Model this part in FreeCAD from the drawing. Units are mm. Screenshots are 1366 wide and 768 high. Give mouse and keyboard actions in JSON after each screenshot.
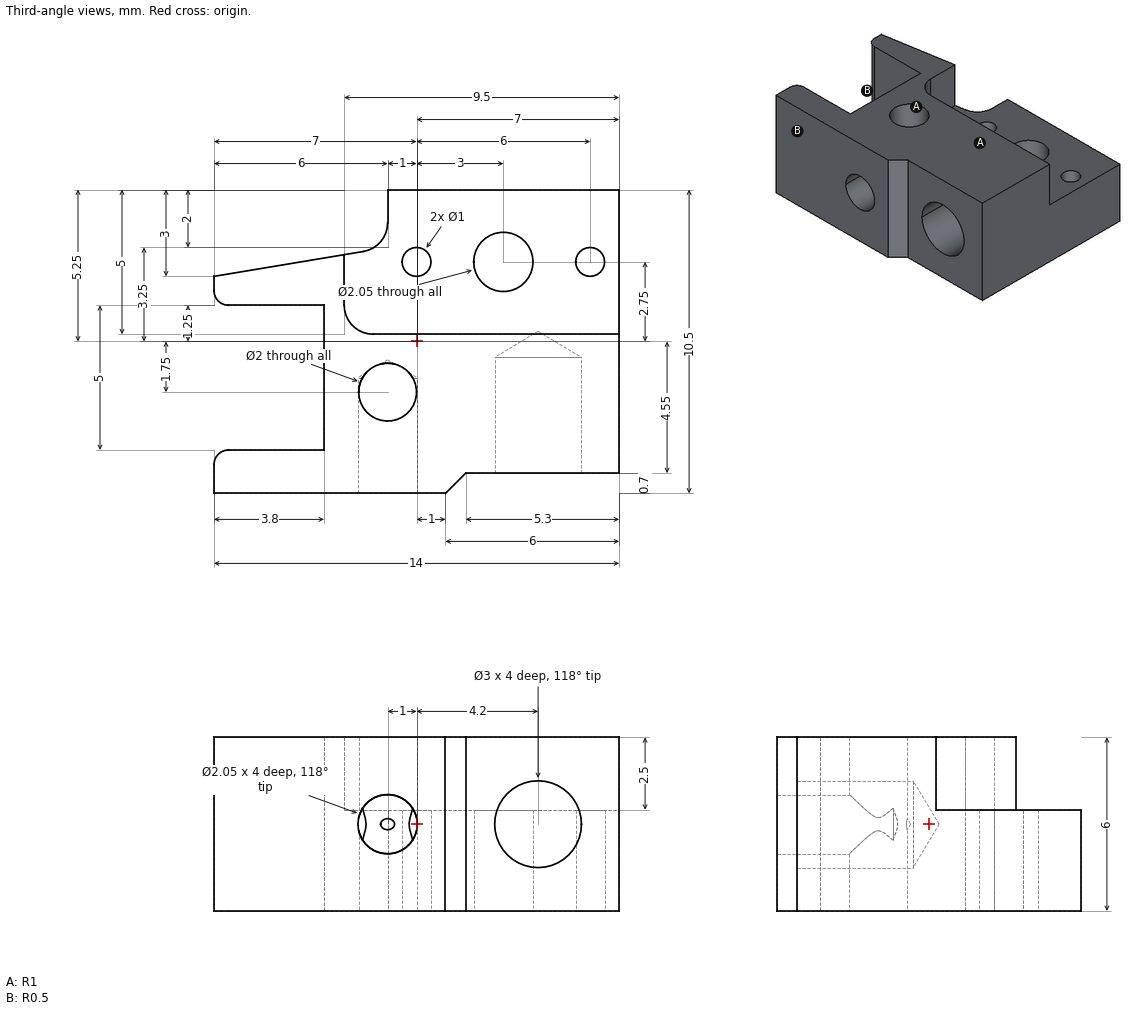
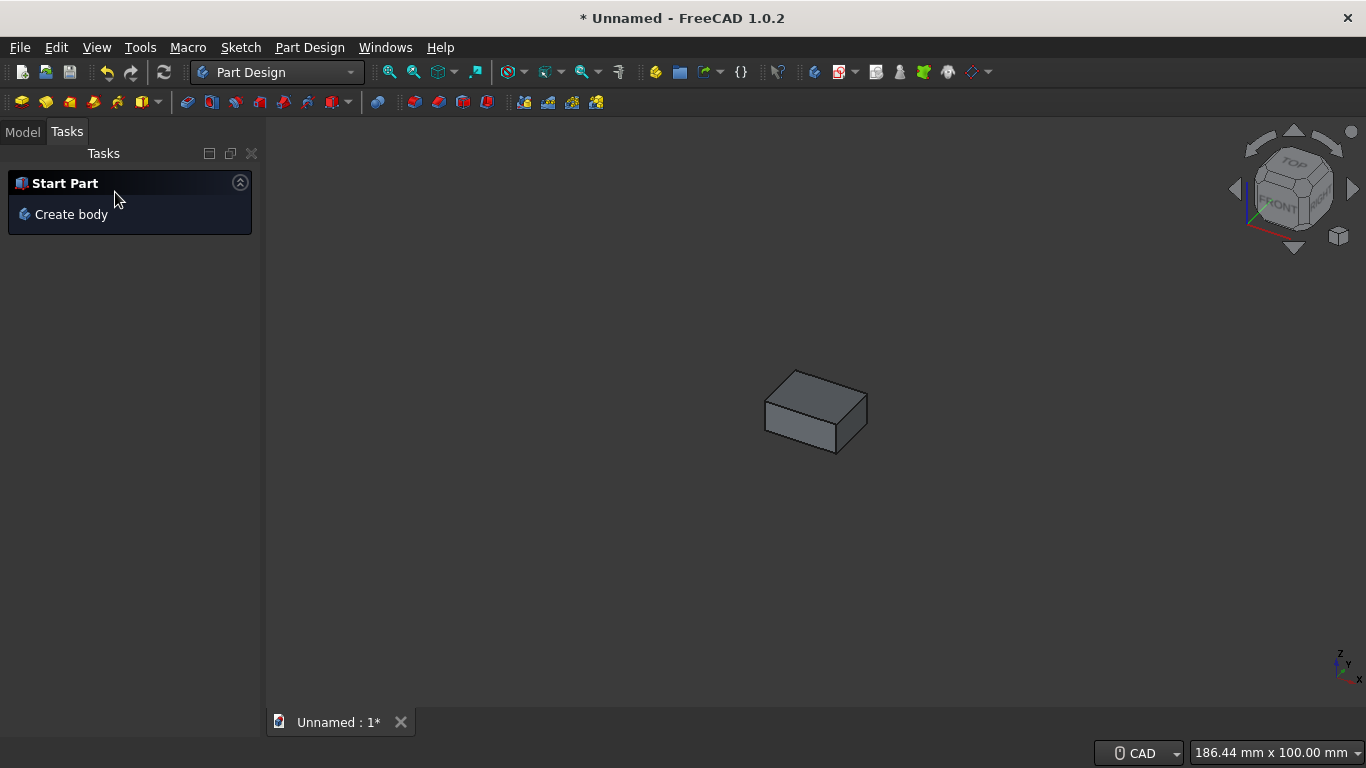
{"action": "left_click", "coordinate": [390, 72]}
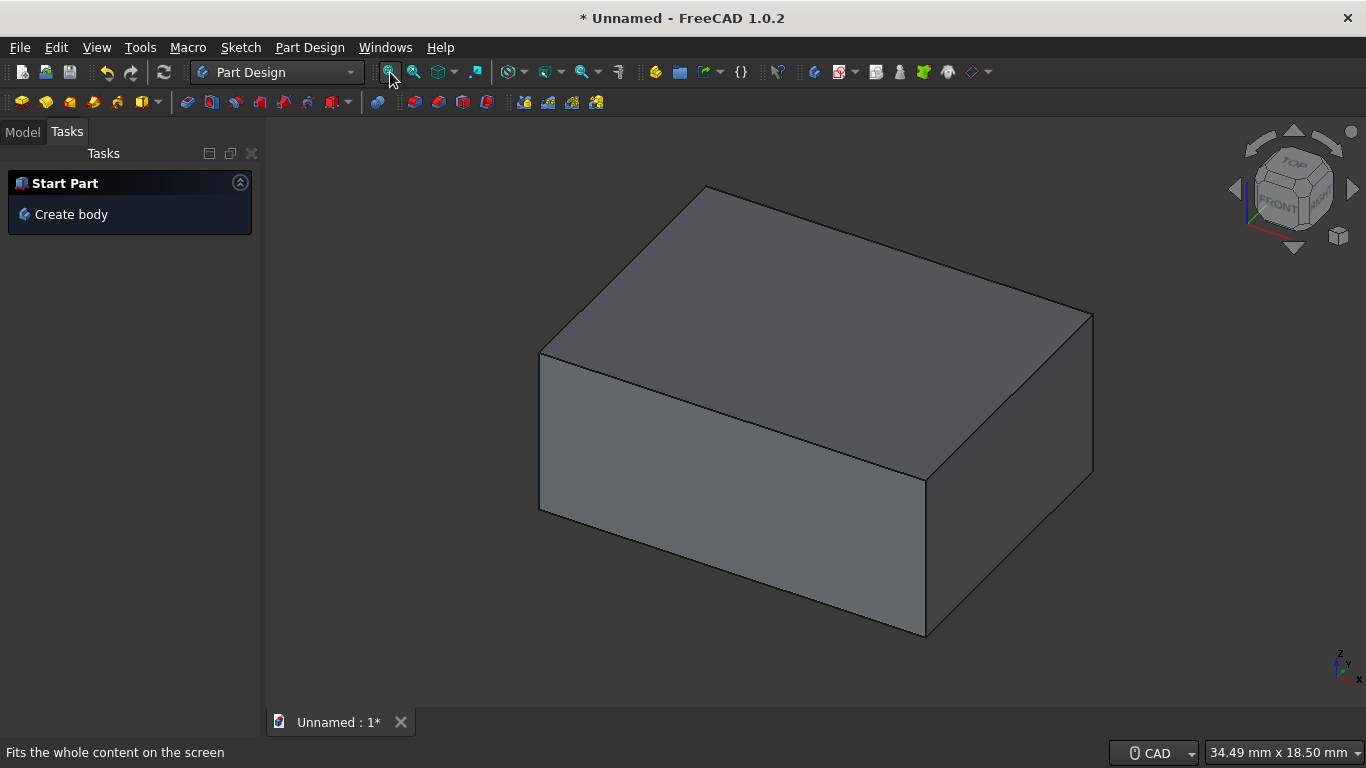
{"action": "left_click", "coordinate": [816, 333]}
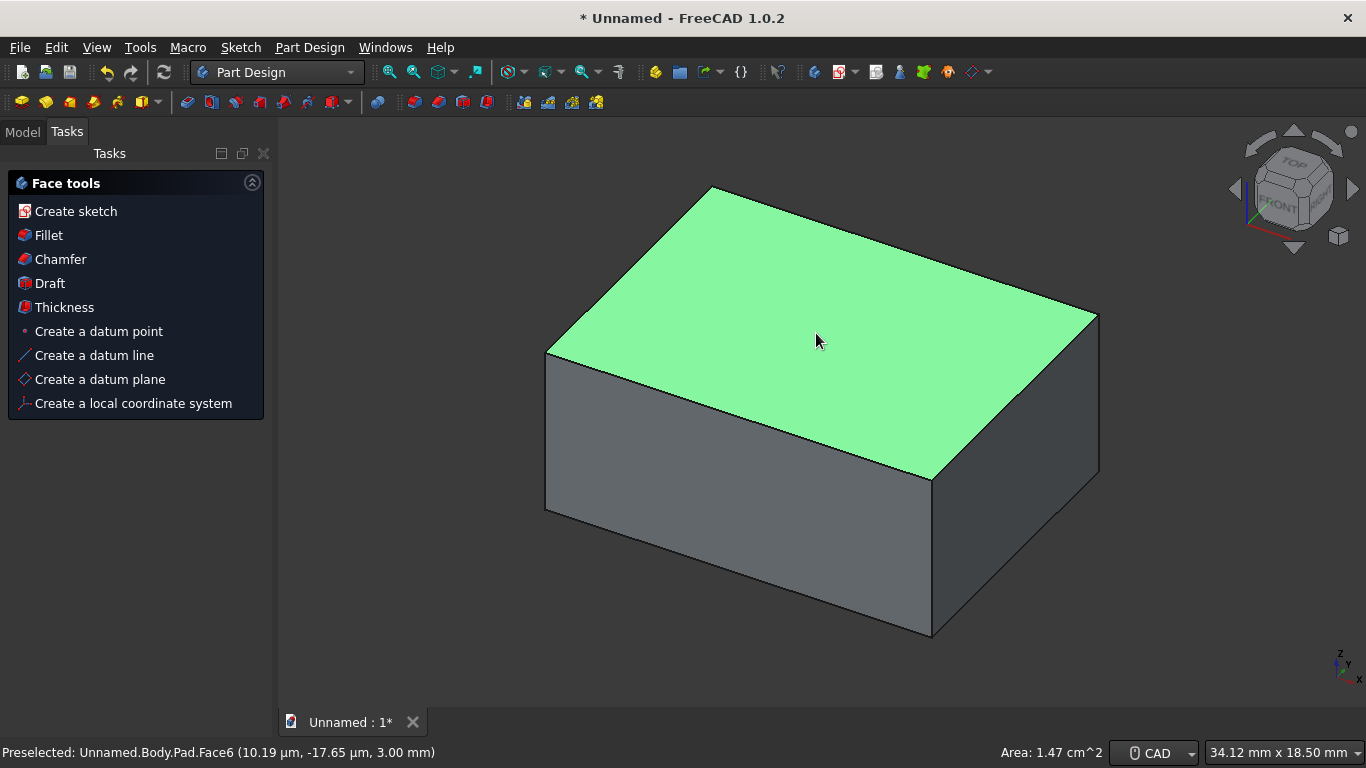
{"action": "left_click", "coordinate": [840, 72]}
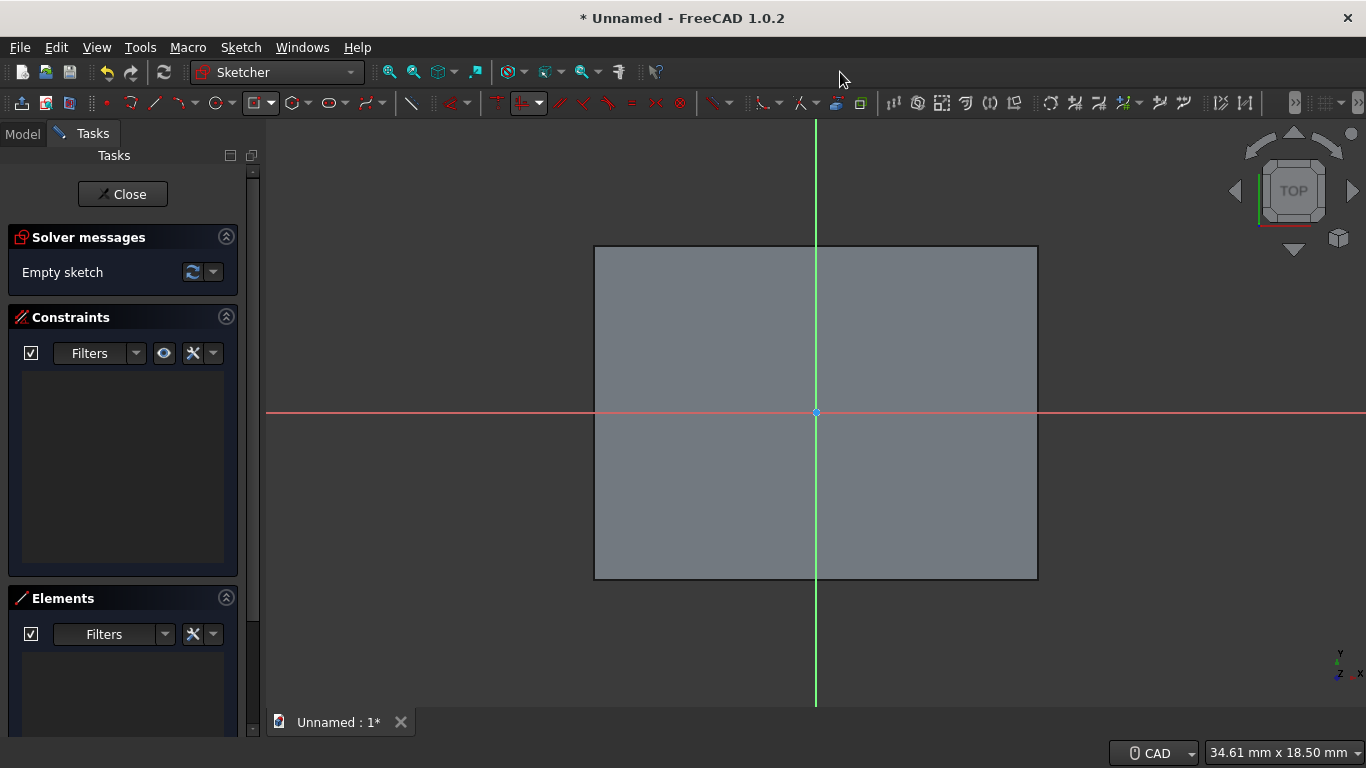
{"action": "scroll", "coordinate": [1002, 261], "scroll_direction": "up", "scroll_amount": 4}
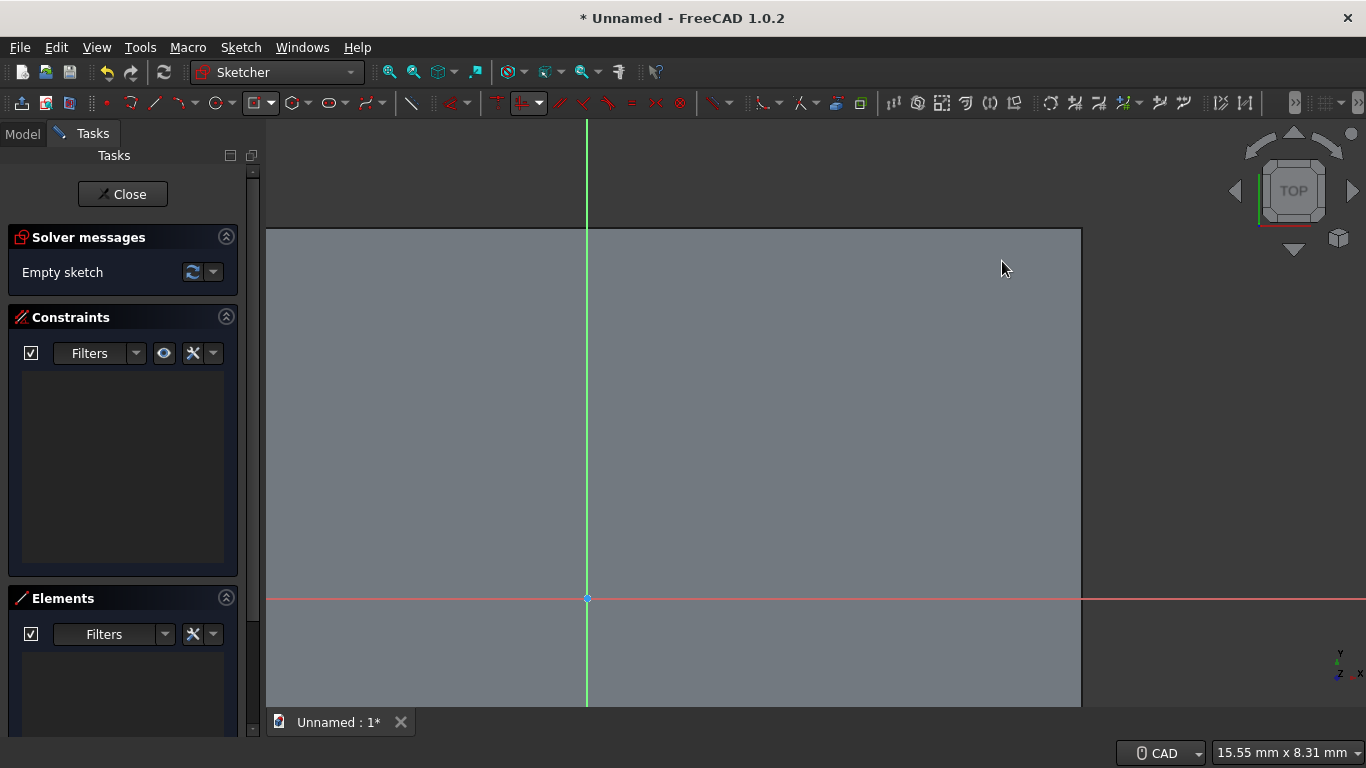
{"action": "left_click", "coordinate": [274, 104]}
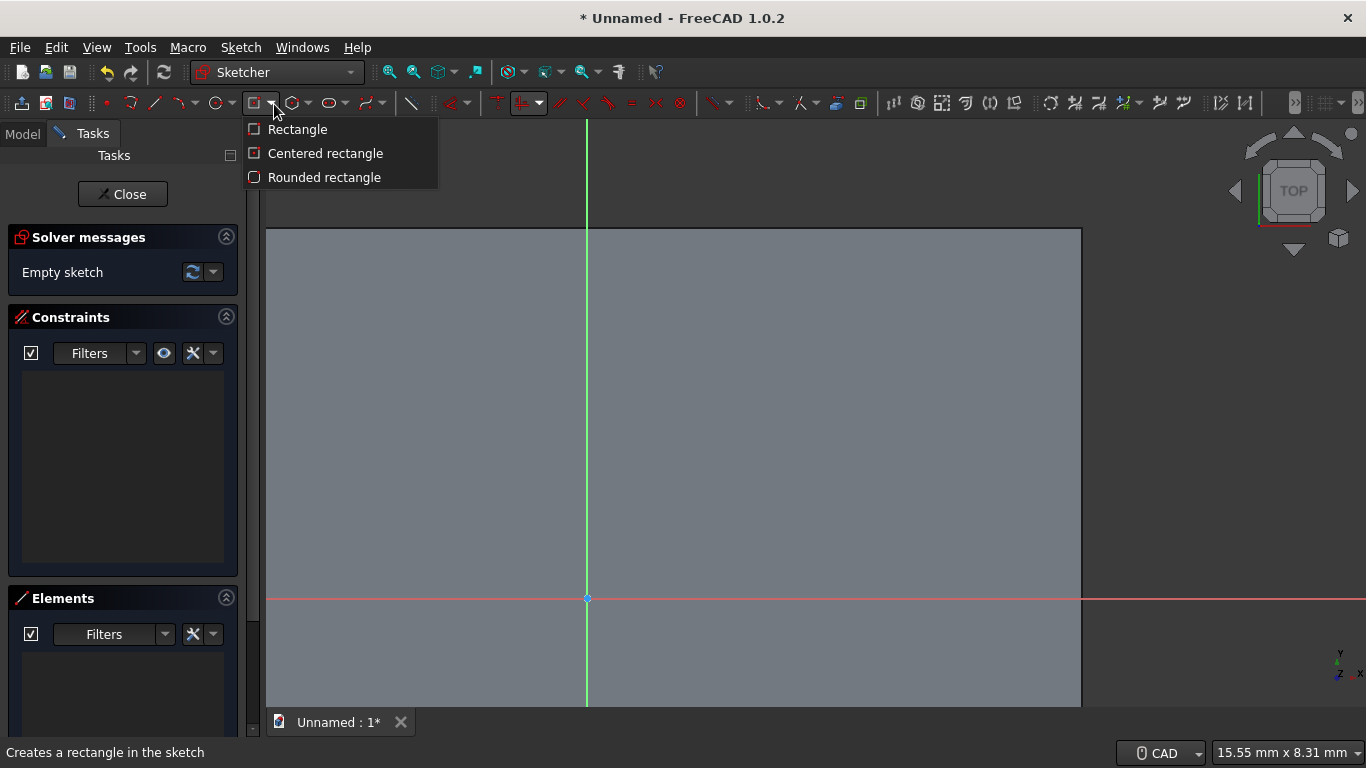
{"action": "left_click", "coordinate": [340, 129]}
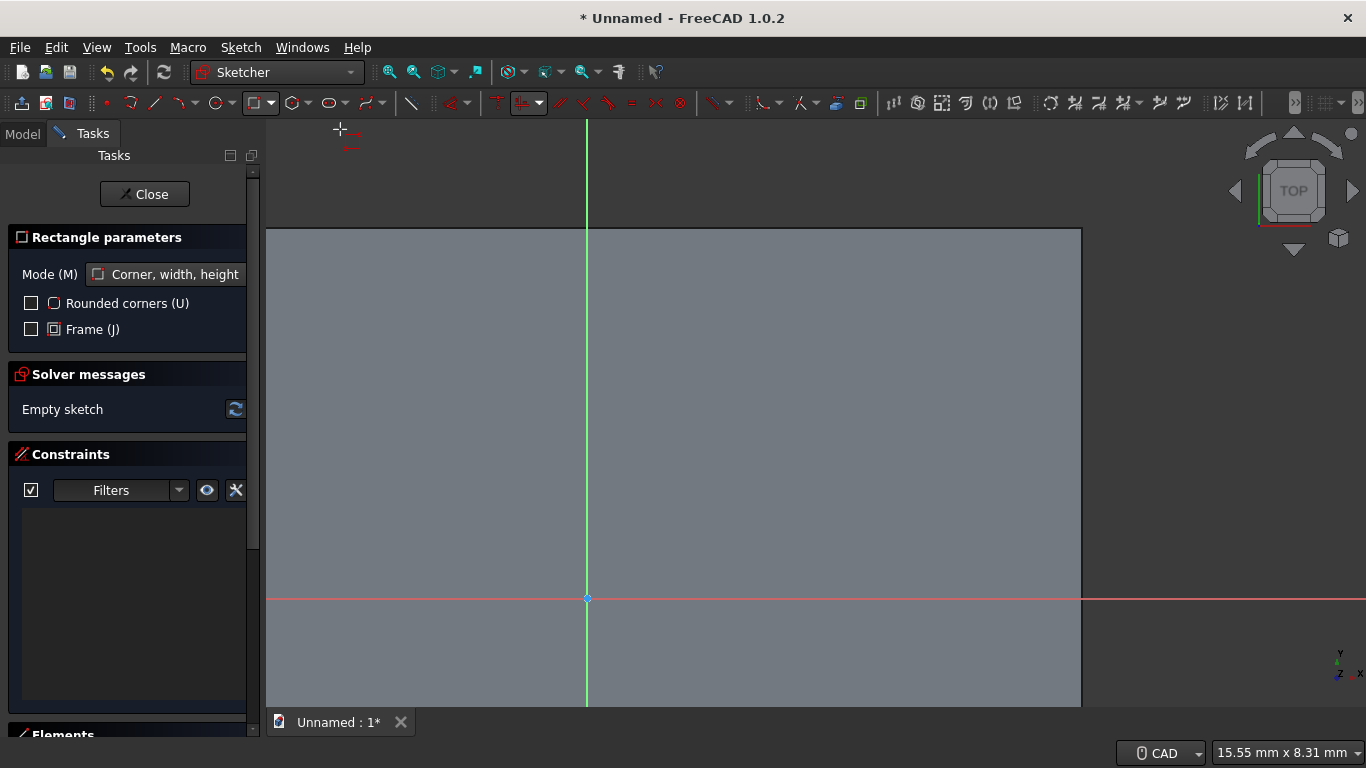
{"action": "left_click", "coordinate": [410, 228]}
{"action": "left_click", "coordinate": [1082, 581]}
{"action": "key", "text": "Escape"}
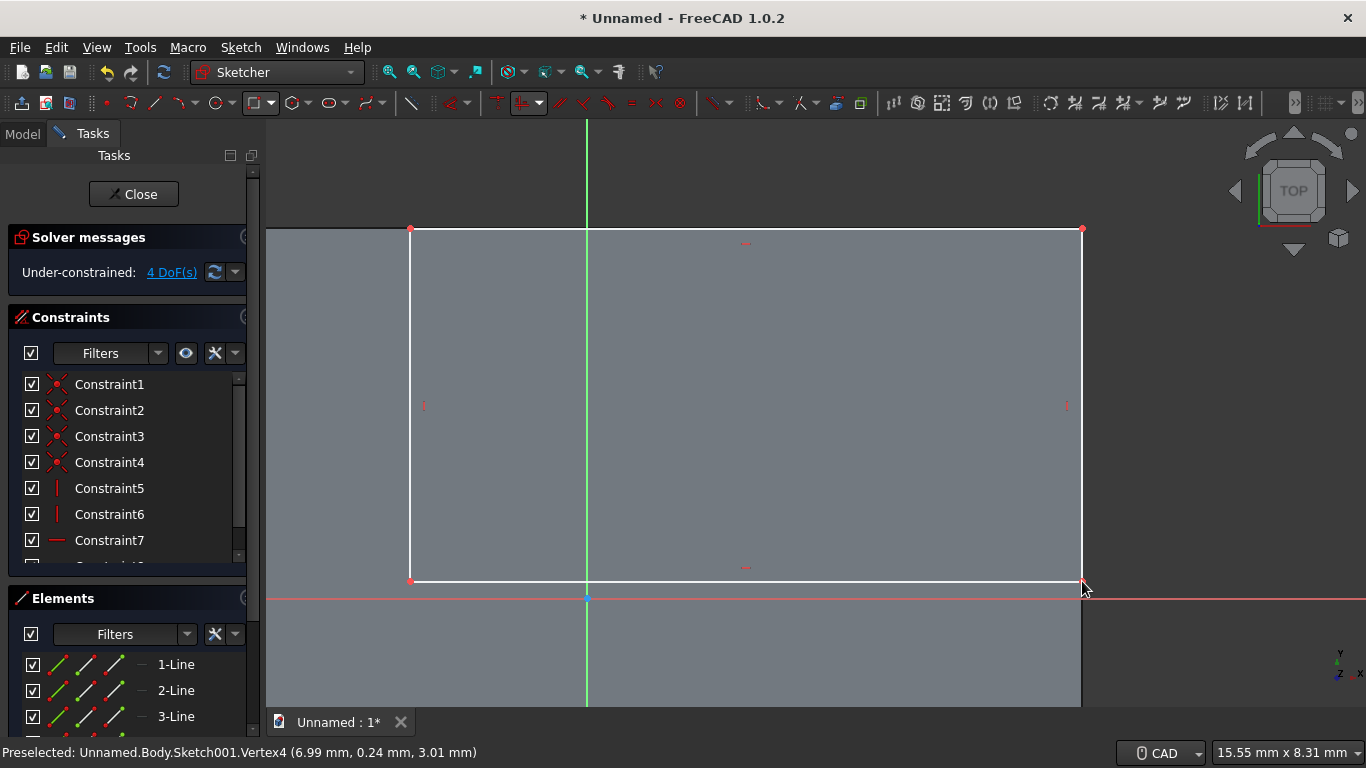
{"action": "left_click", "coordinate": [450, 104]}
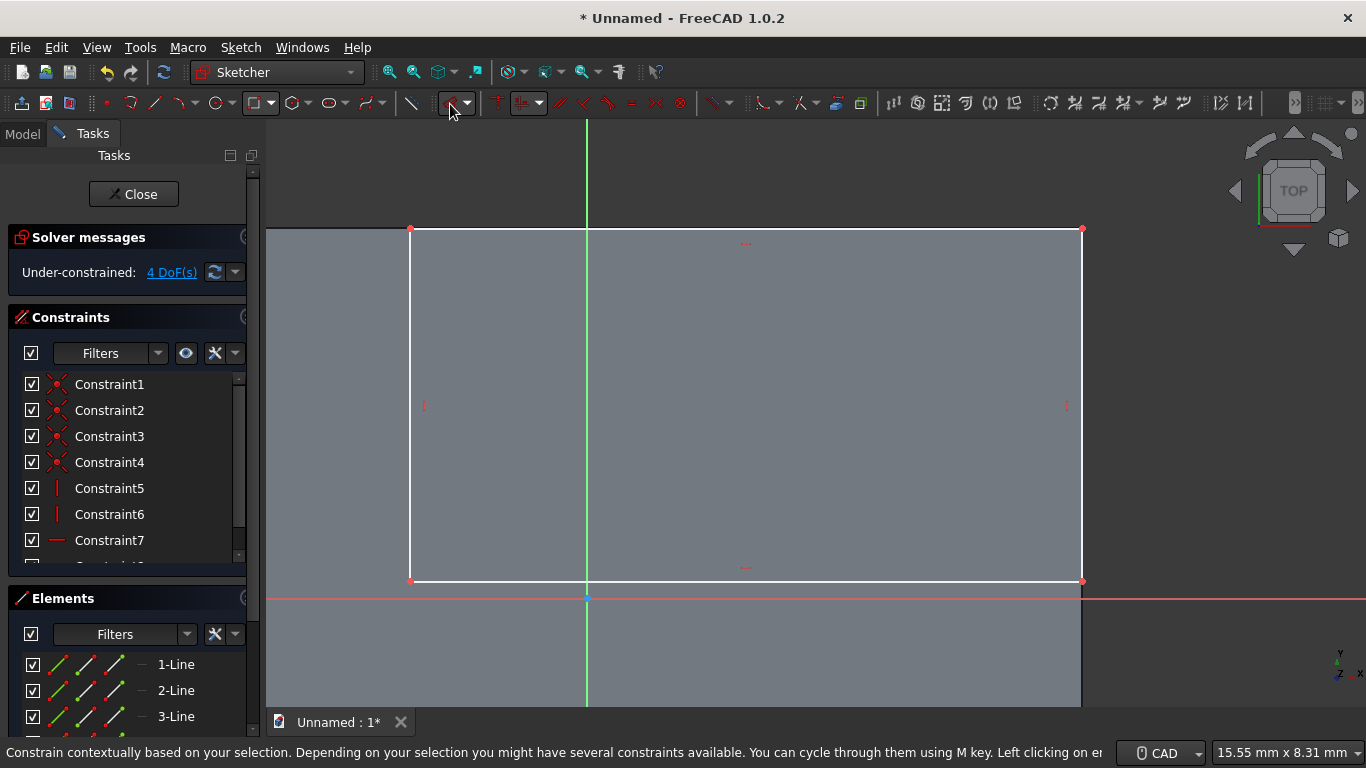
{"action": "left_click", "coordinate": [410, 335]}
{"action": "left_click", "coordinate": [376, 406]}